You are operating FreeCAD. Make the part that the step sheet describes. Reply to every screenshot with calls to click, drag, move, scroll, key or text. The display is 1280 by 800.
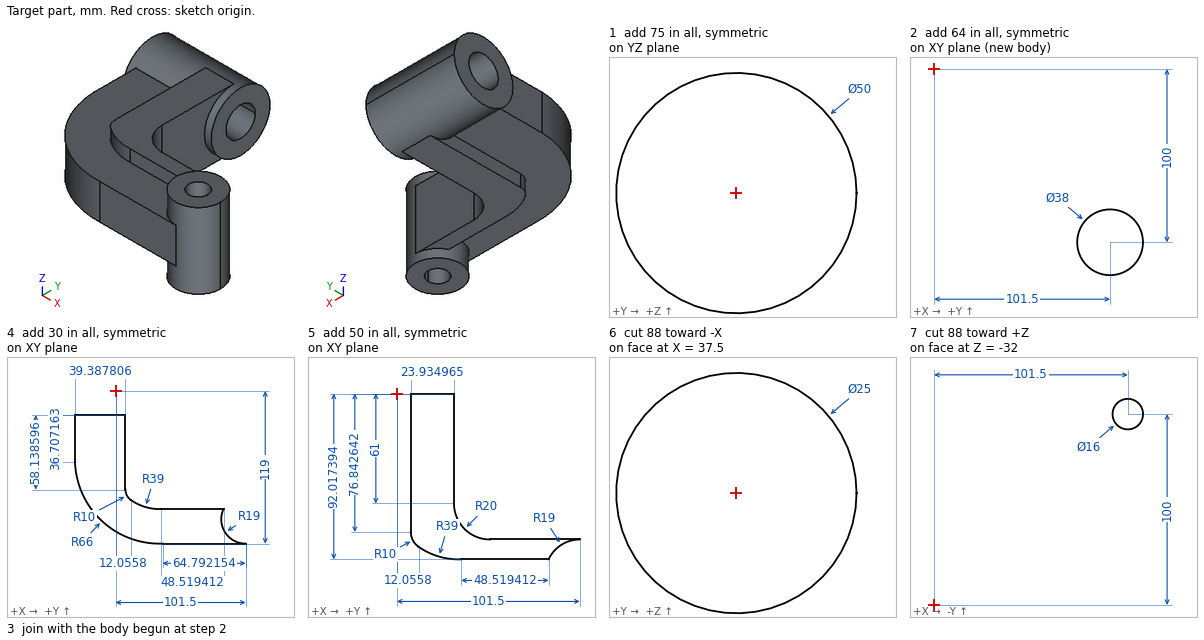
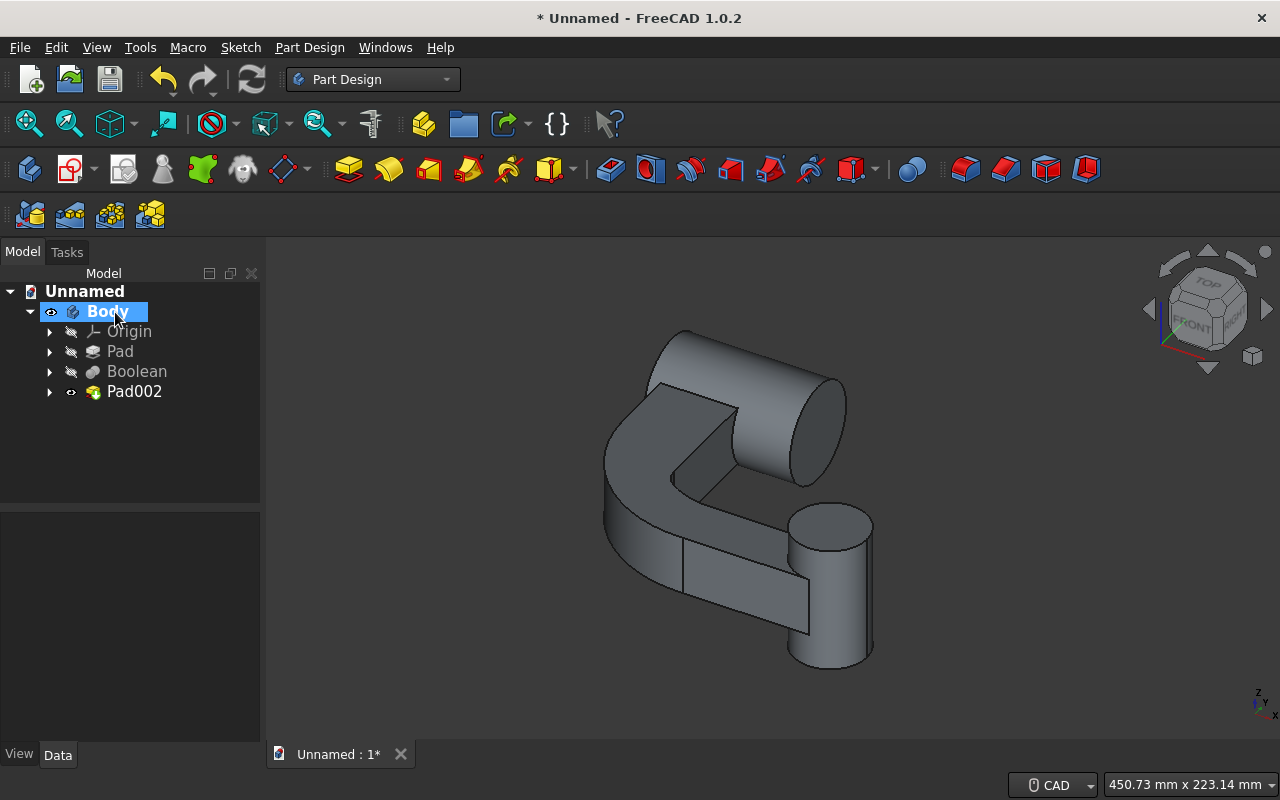
click(70, 170)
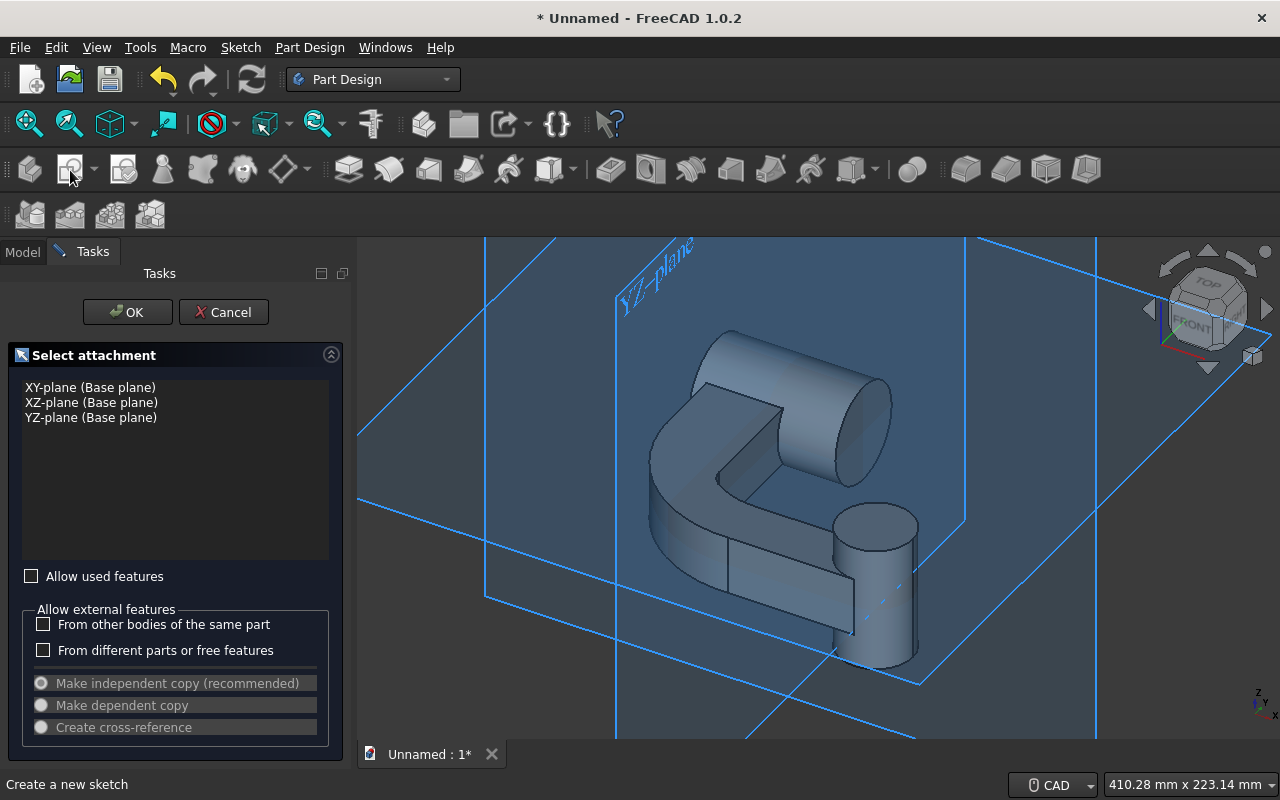
click(82, 388)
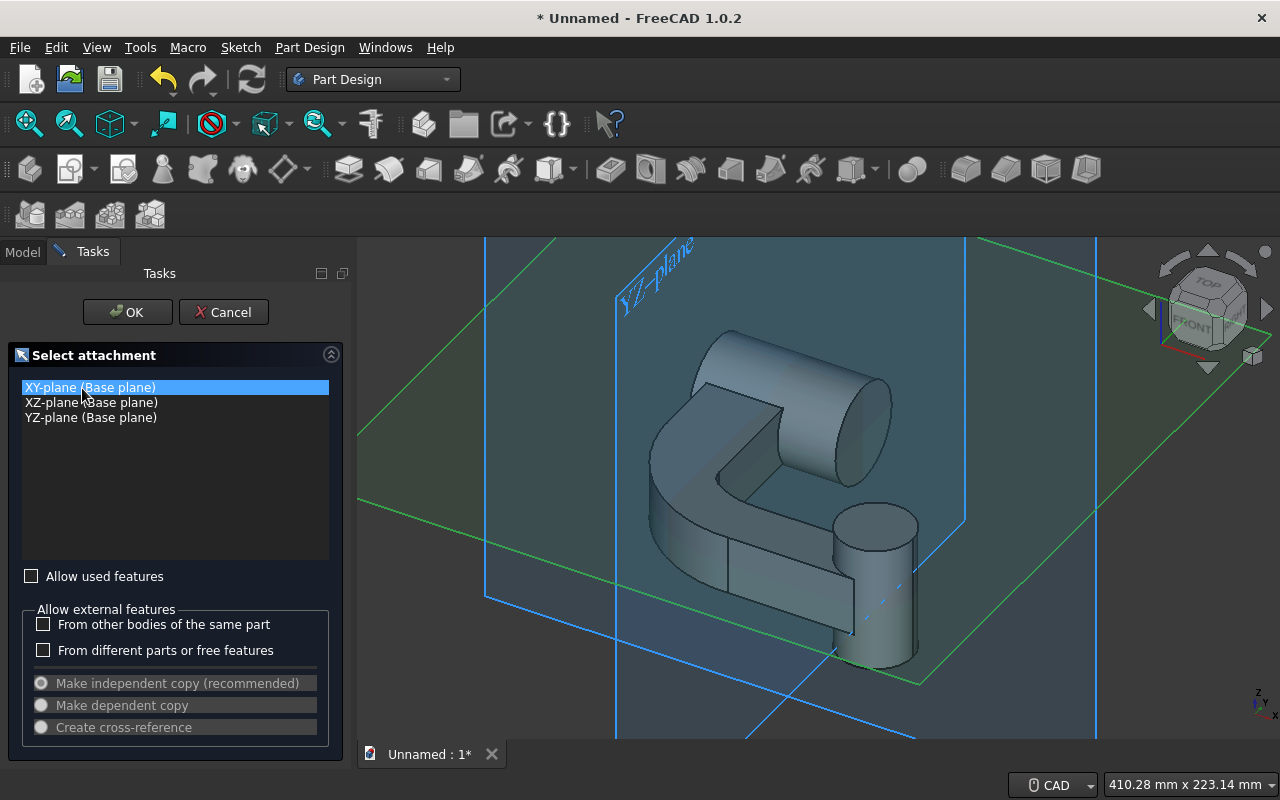
click(128, 312)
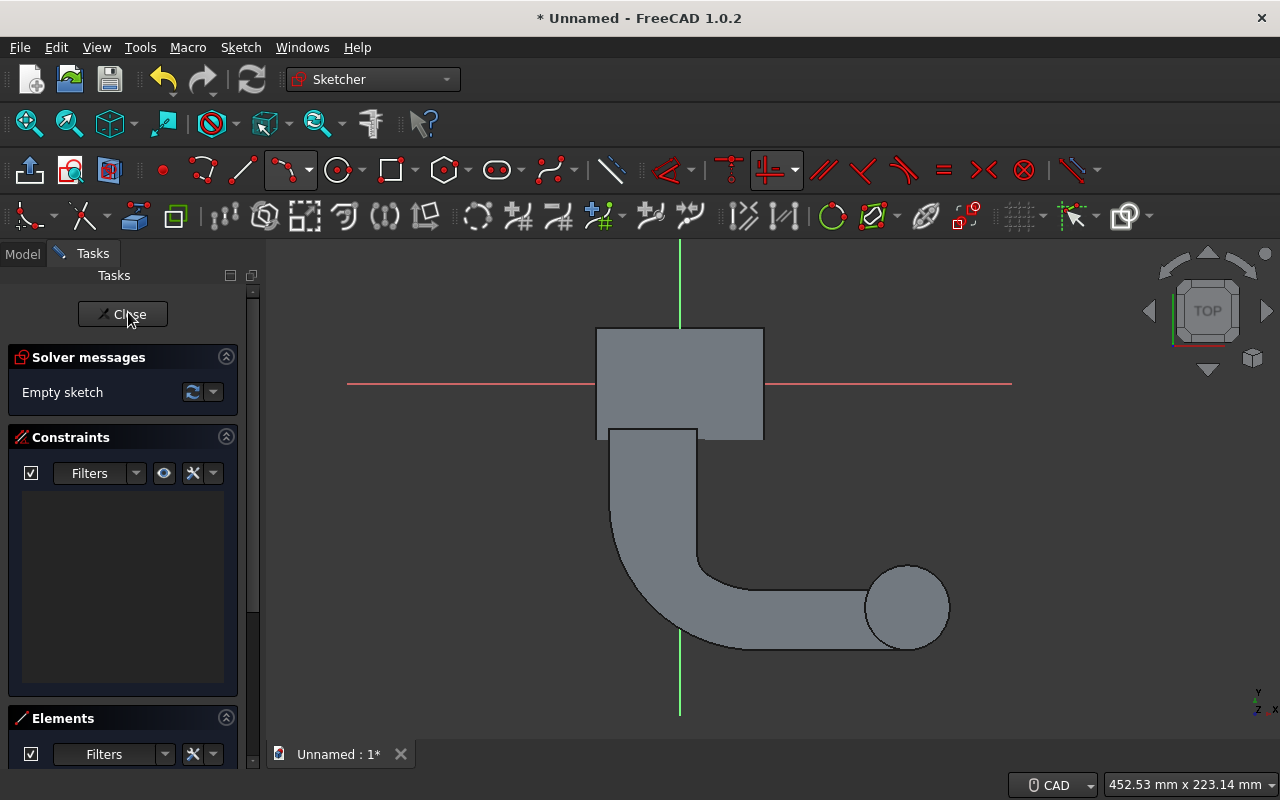
click(110, 170)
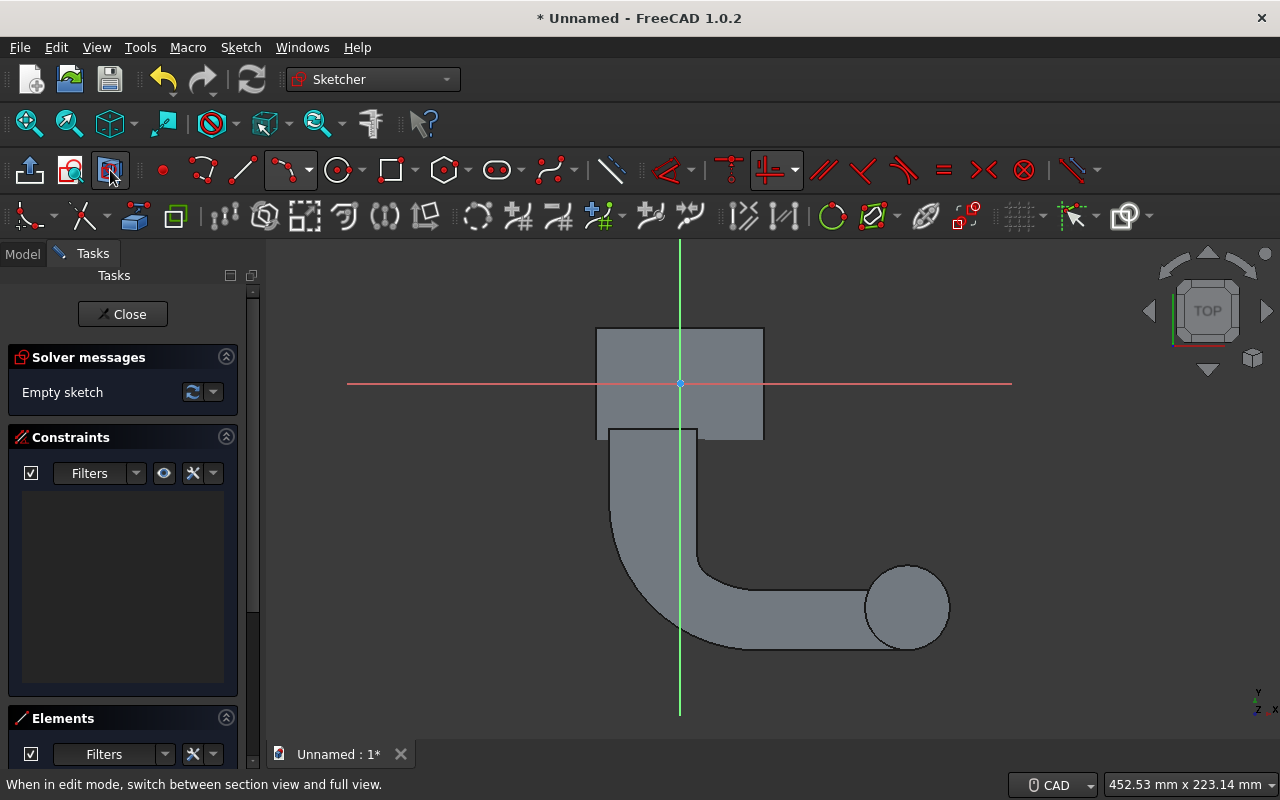
scroll(975, 482, up, 2)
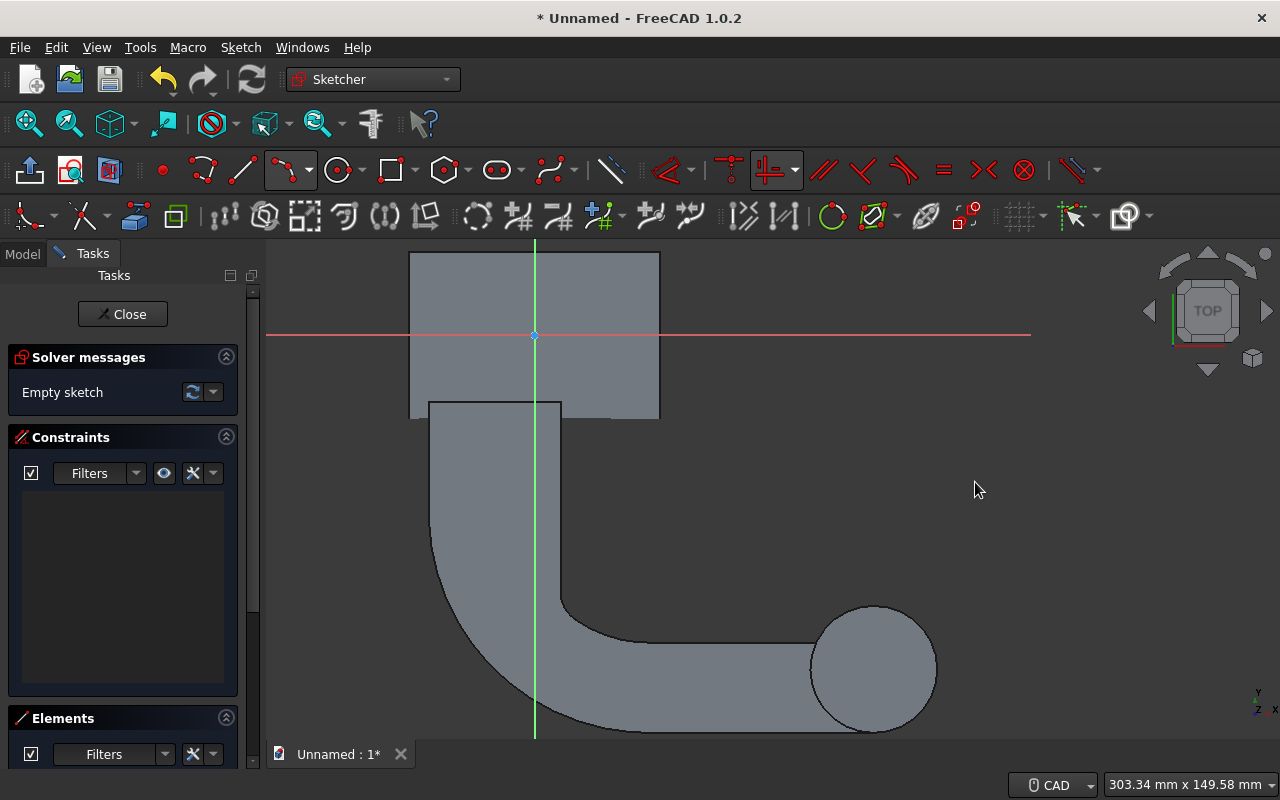
click(204, 170)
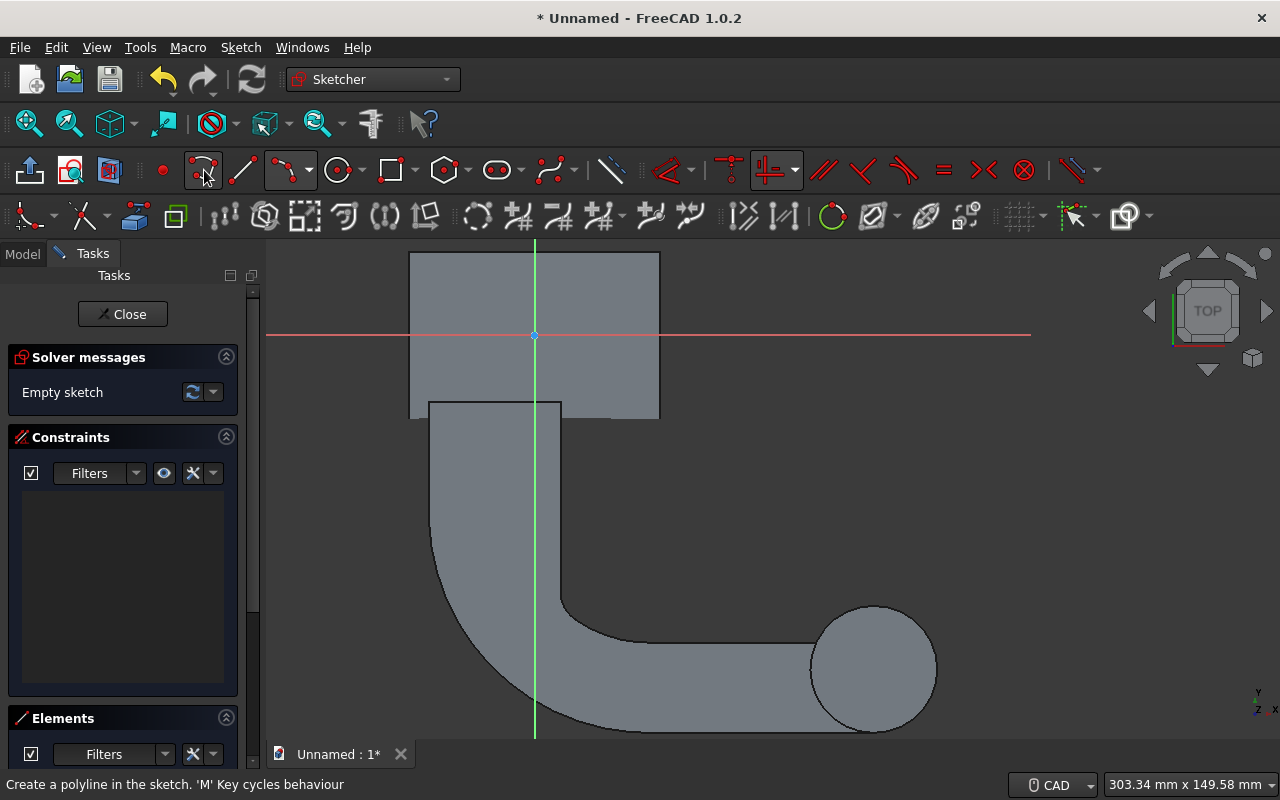
click(641, 539)
click(641, 335)
click(561, 344)
click(561, 592)
right_click(561, 592)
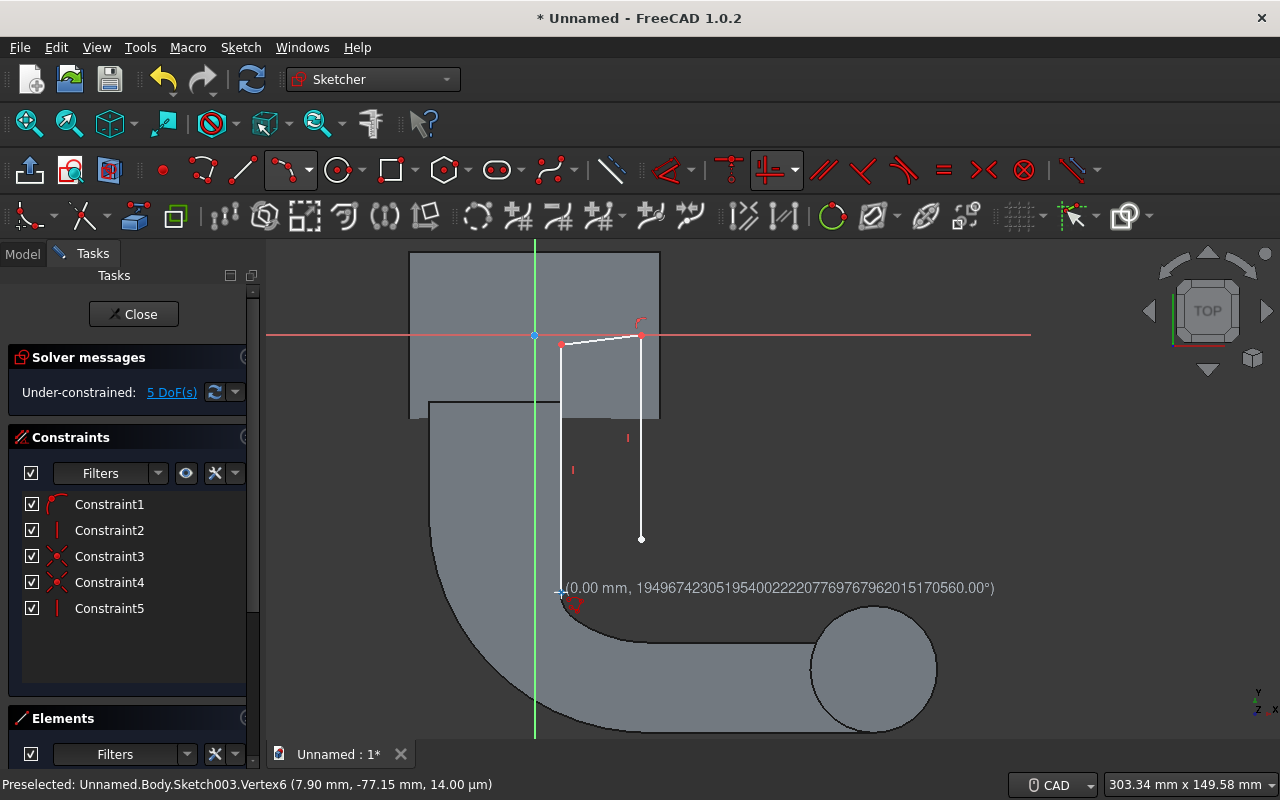
click(244, 170)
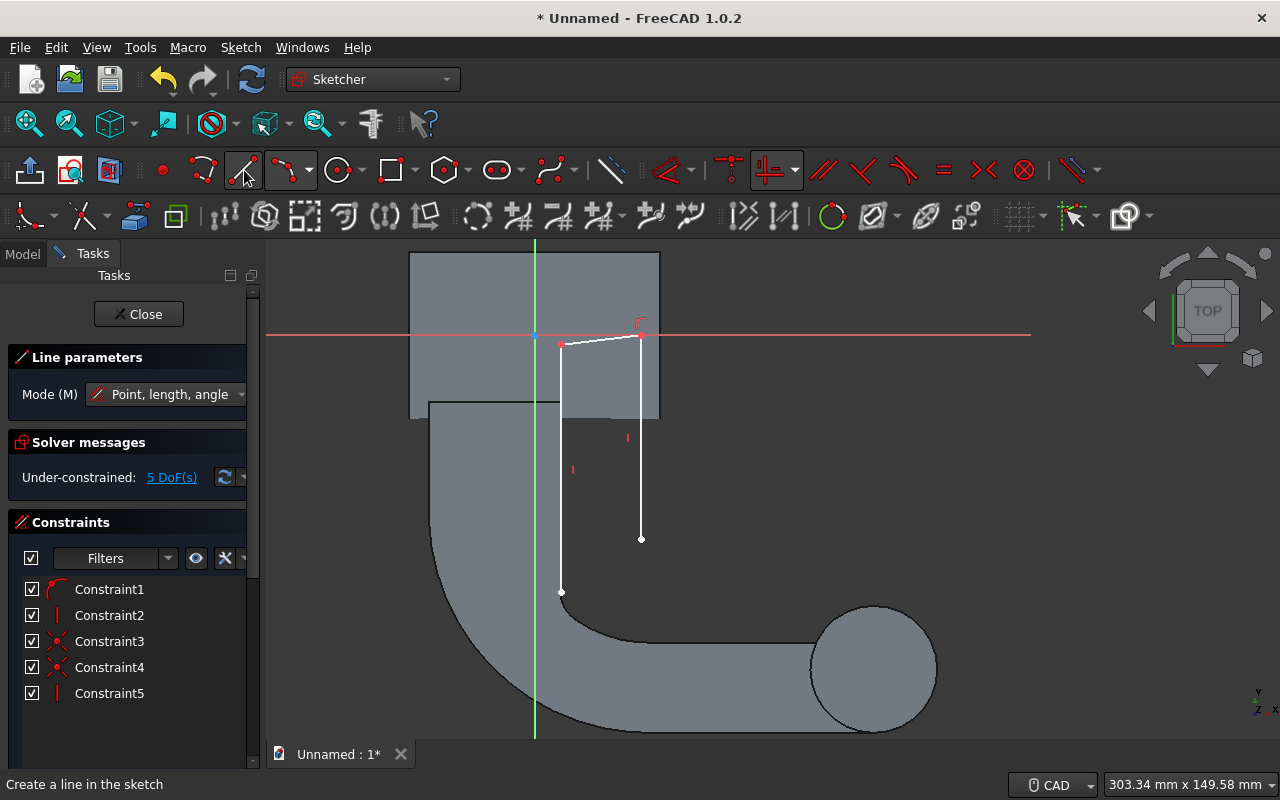
click(654, 643)
click(816, 643)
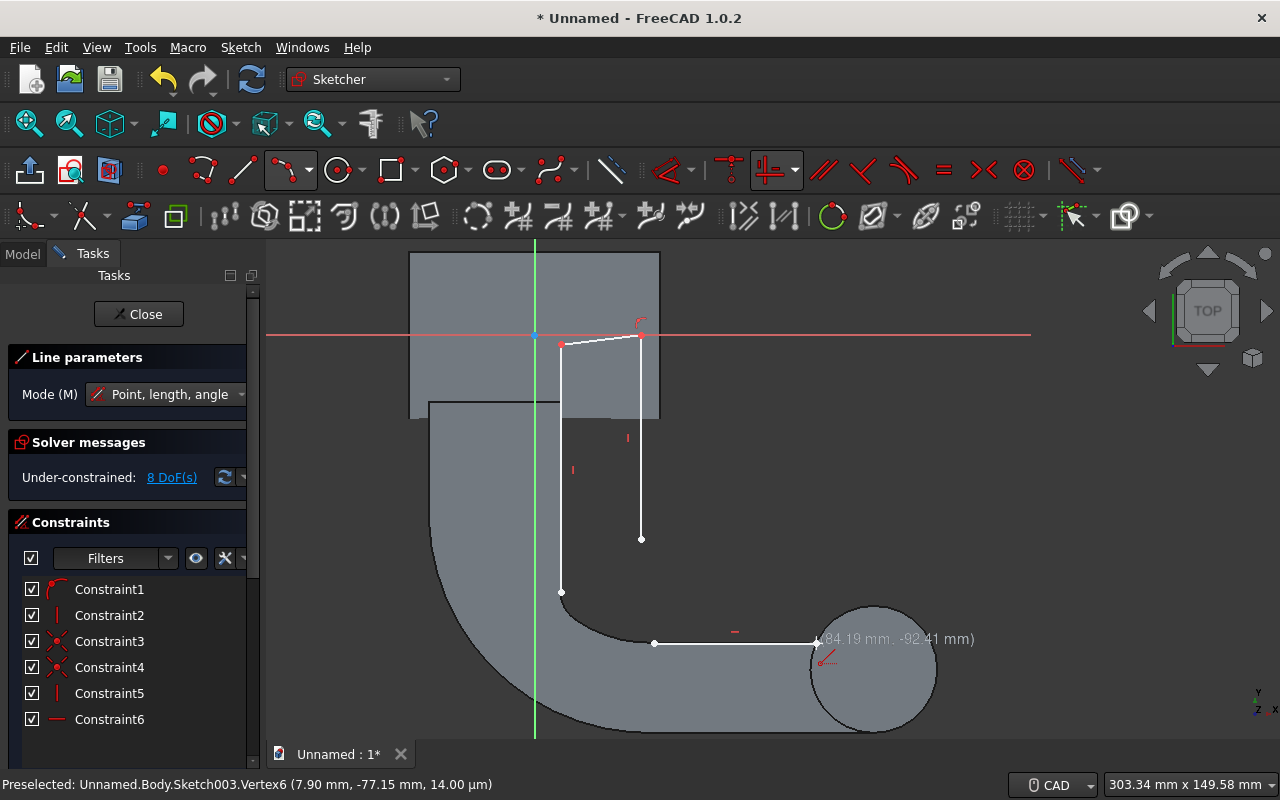
click(874, 606)
click(707, 606)